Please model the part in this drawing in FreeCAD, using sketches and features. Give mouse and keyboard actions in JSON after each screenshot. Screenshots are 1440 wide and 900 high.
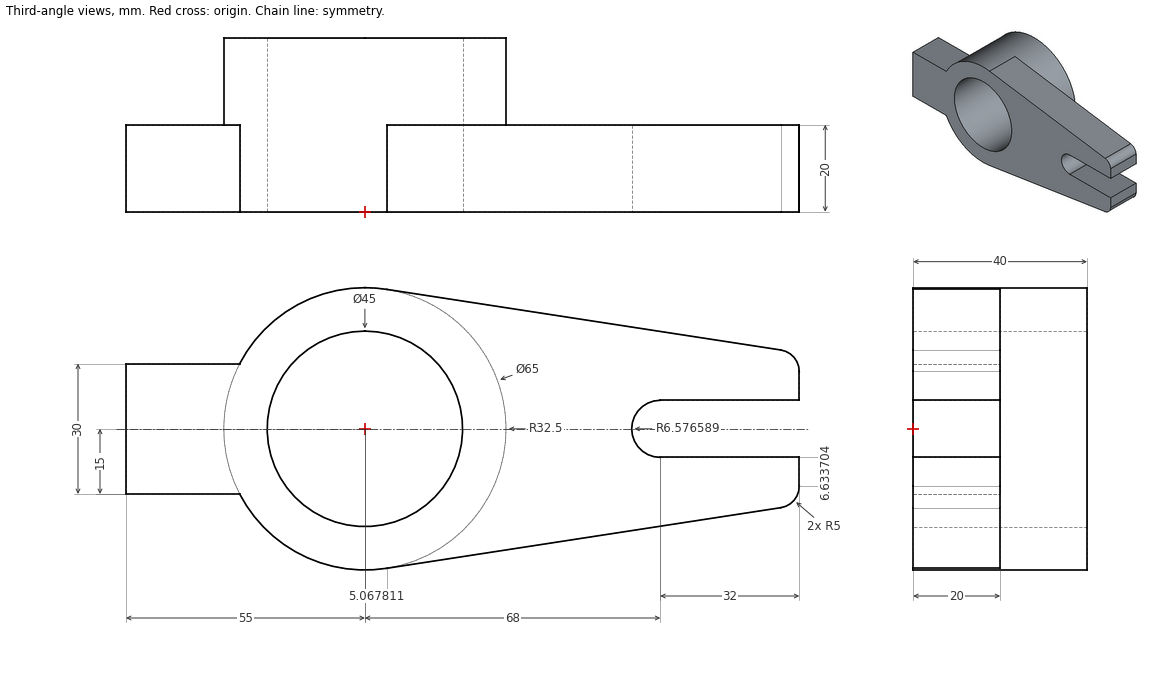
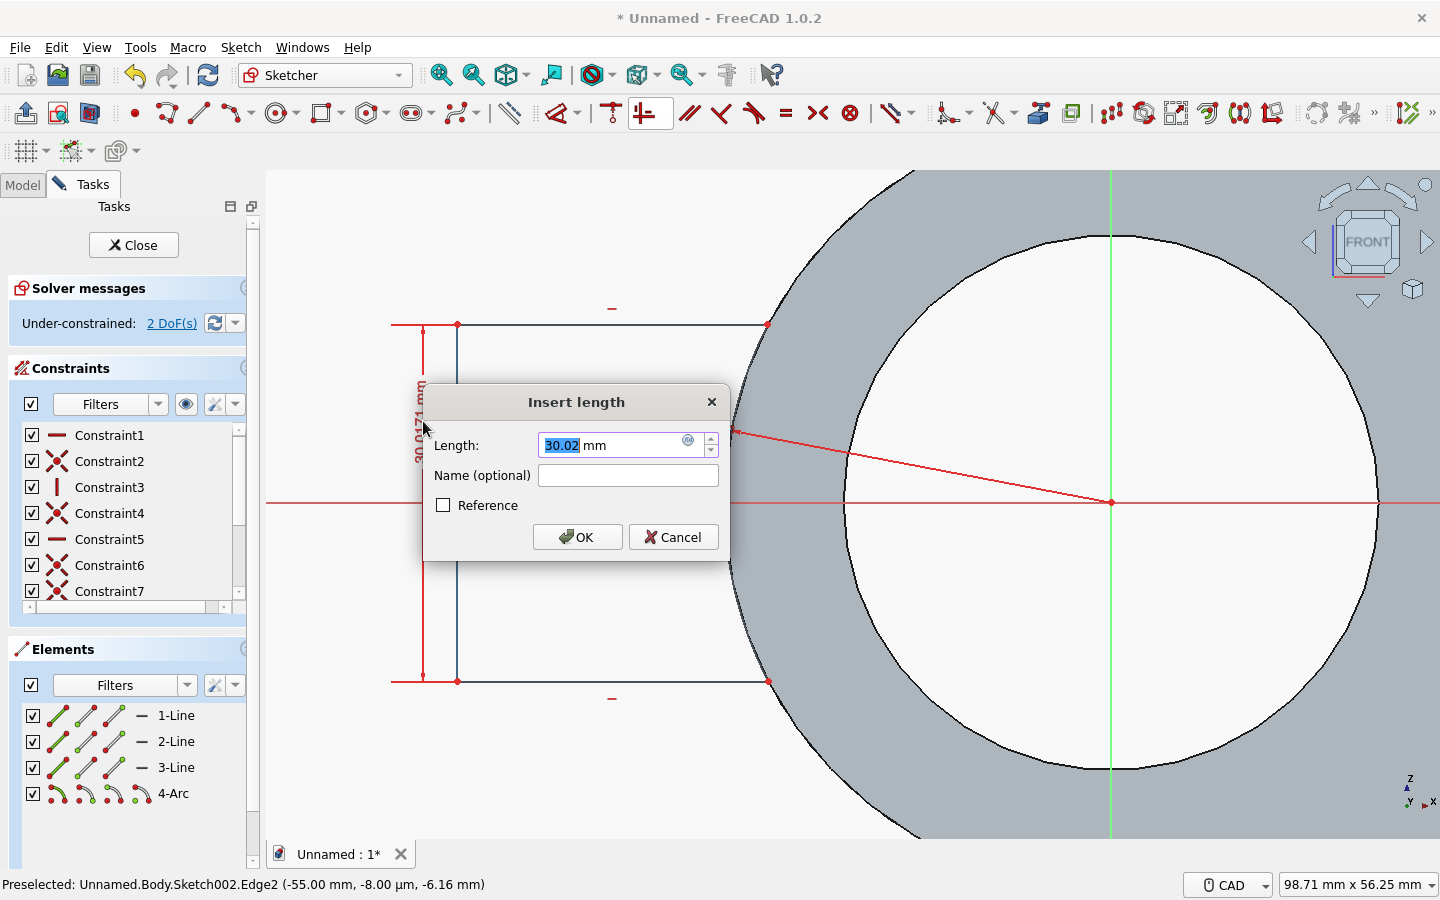
{"action": "type", "text": "30"}
{"action": "key", "text": "Return"}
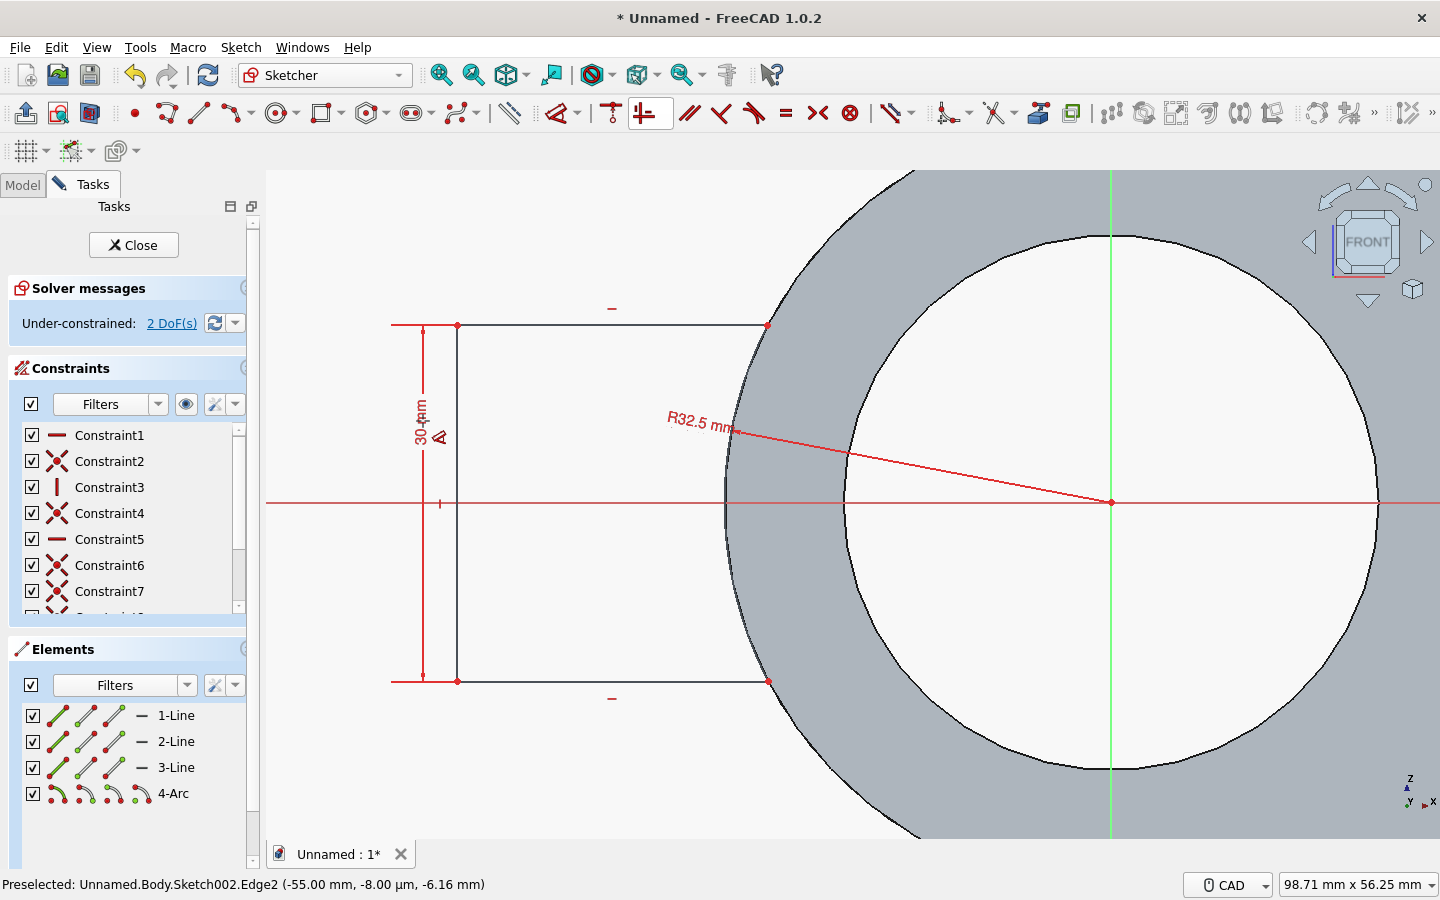
{"action": "left_click", "coordinate": [769, 682]}
{"action": "left_click", "coordinate": [1145, 592]}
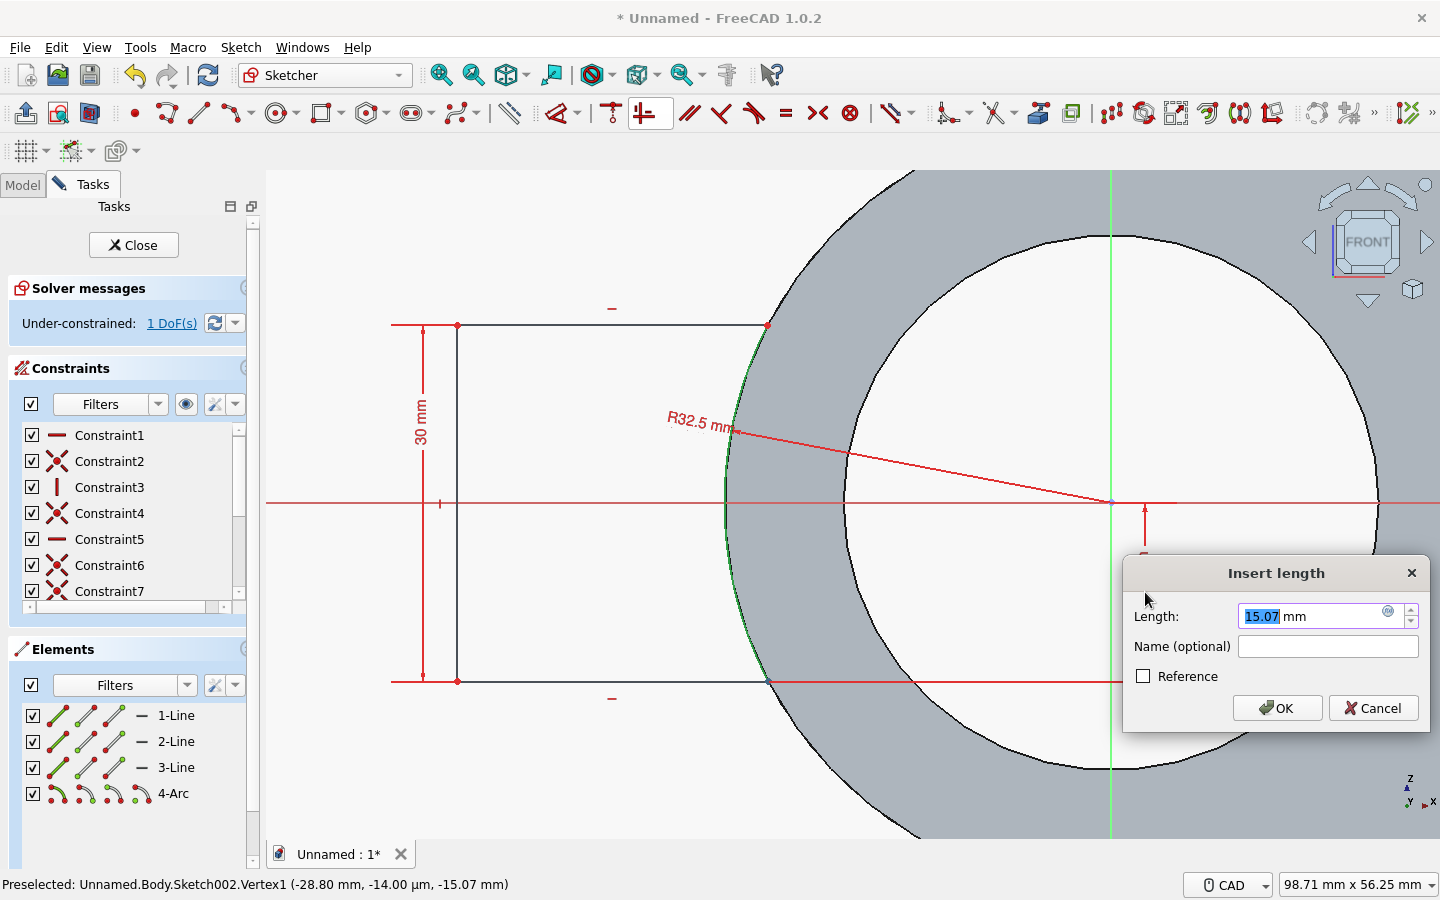
{"action": "type", "text": "15"}
{"action": "key", "text": "Return"}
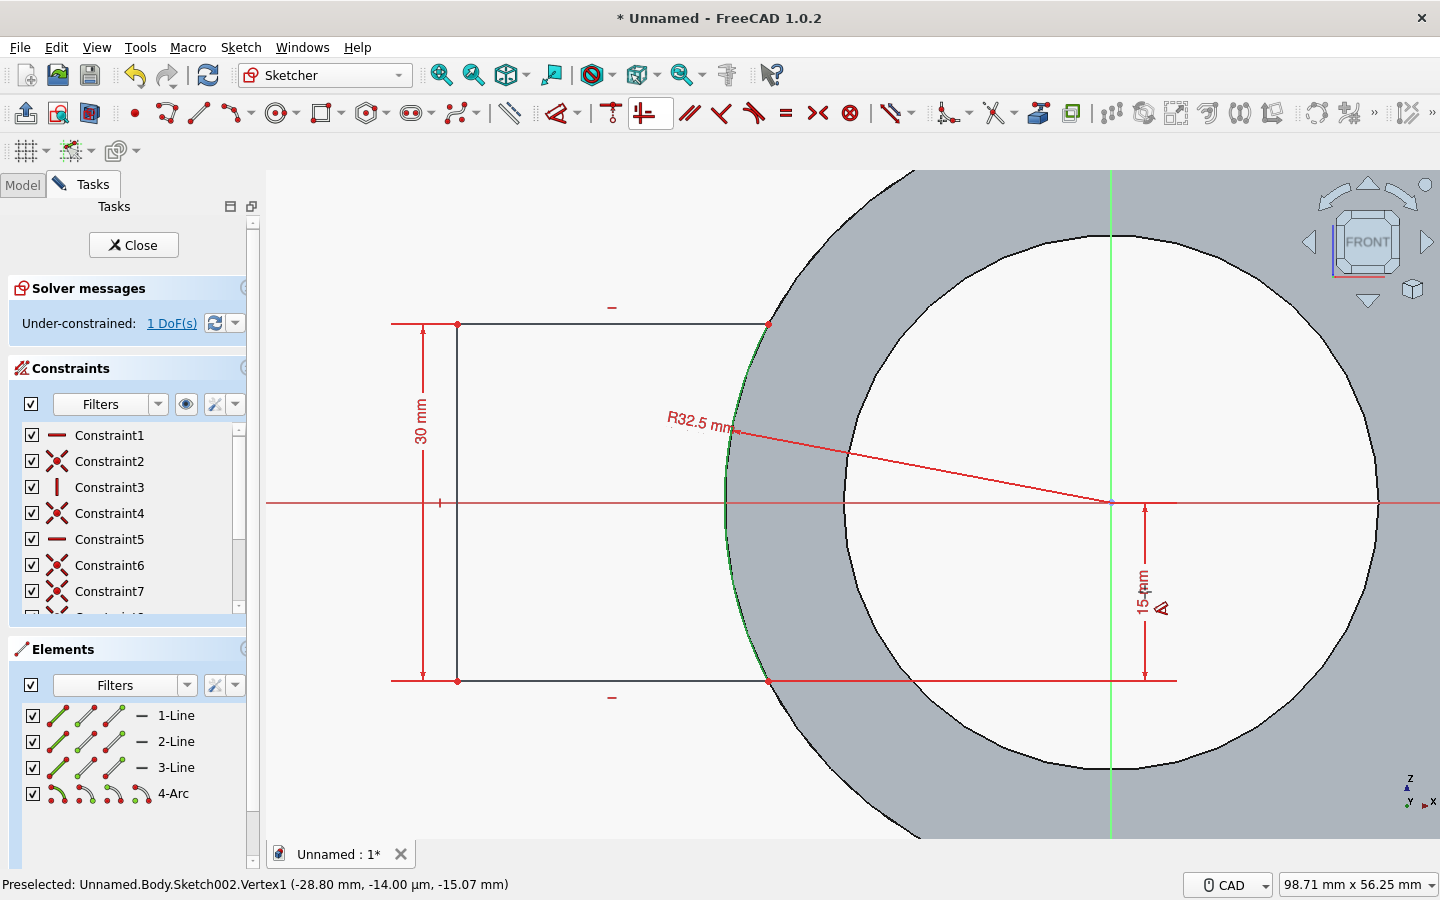
{"action": "left_click", "coordinate": [457, 681]}
{"action": "left_click", "coordinate": [784, 715]}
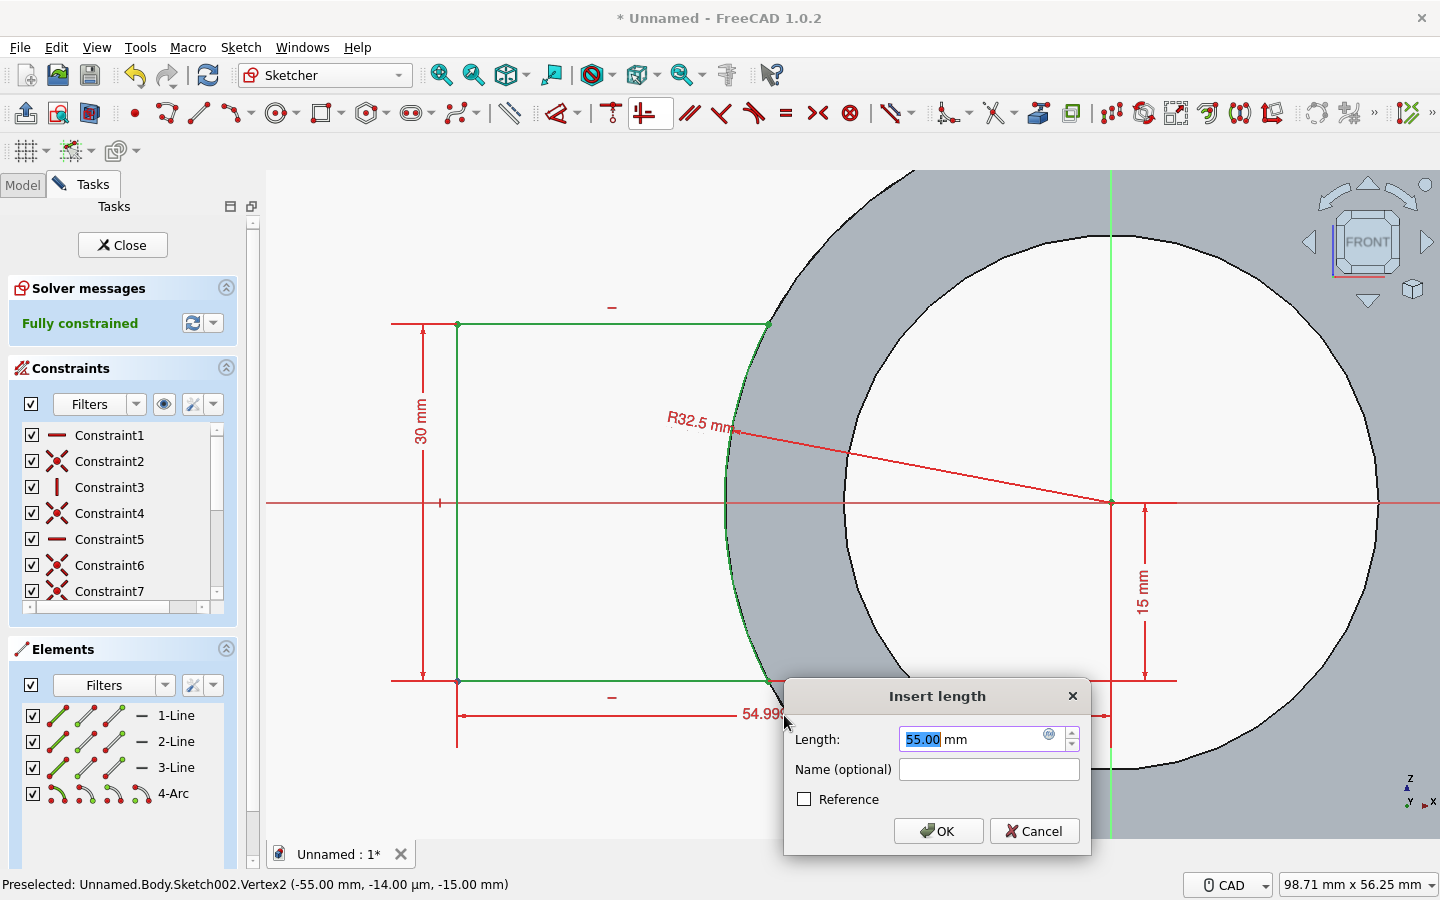
{"action": "type", "text": "55"}
{"action": "key", "text": "Return"}
{"action": "key", "text": "Escape"}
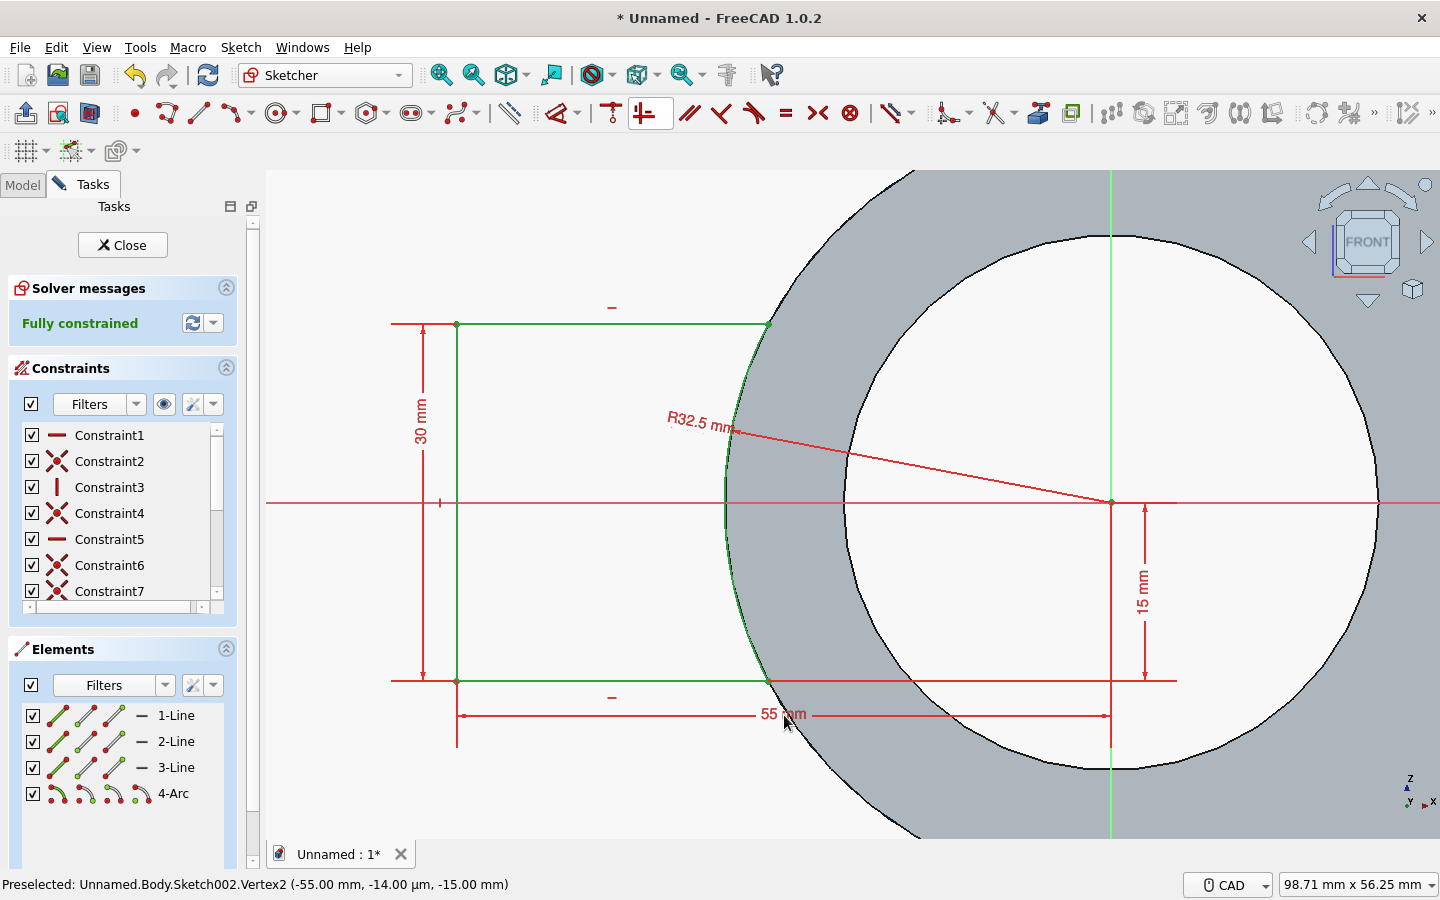
{"action": "left_click", "coordinate": [123, 245]}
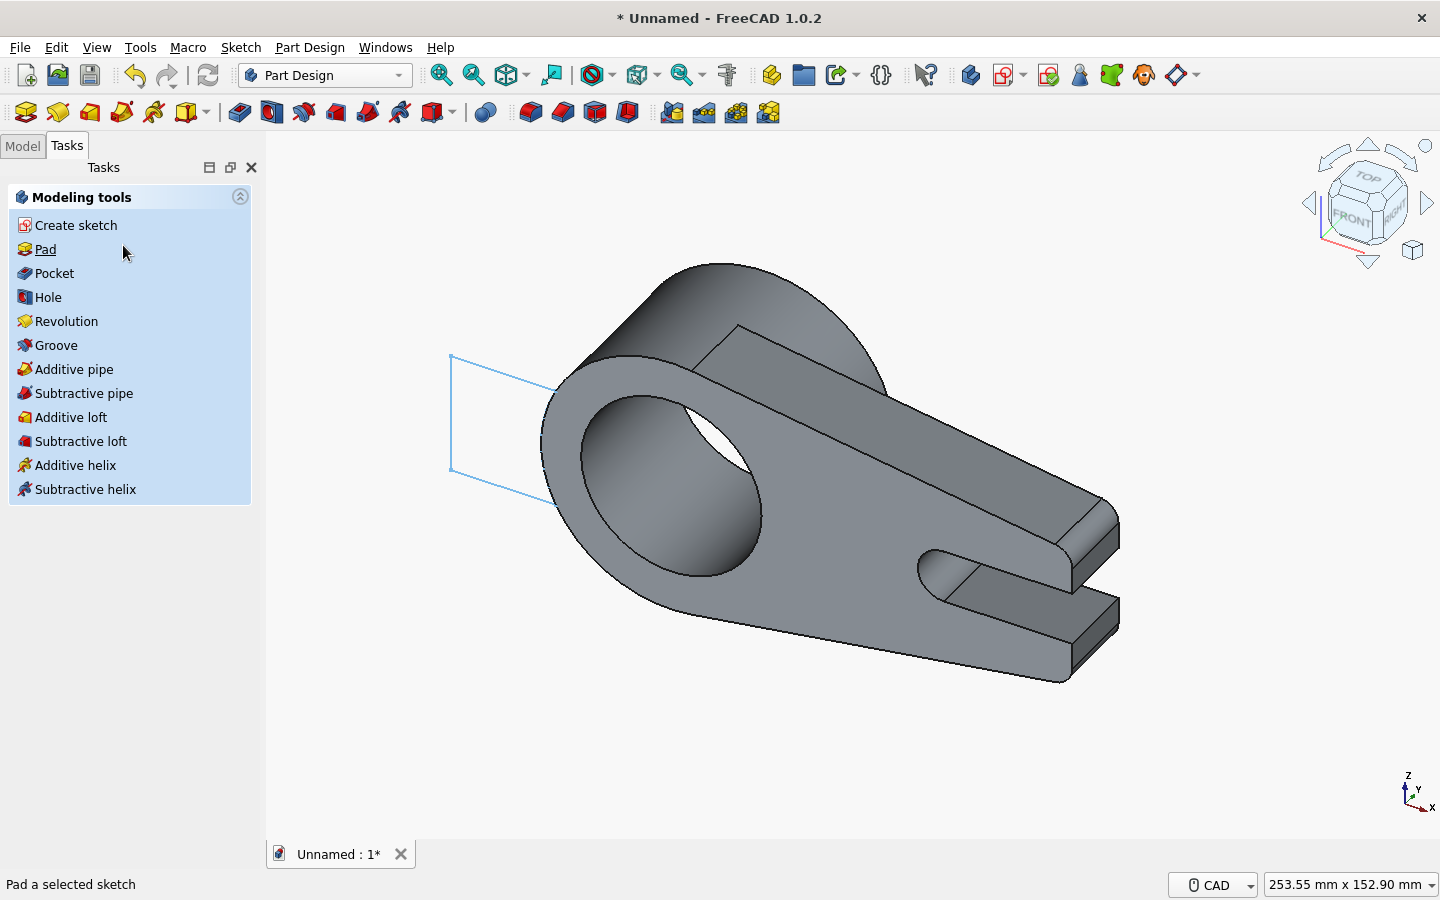
{"action": "left_click", "coordinate": [26, 112]}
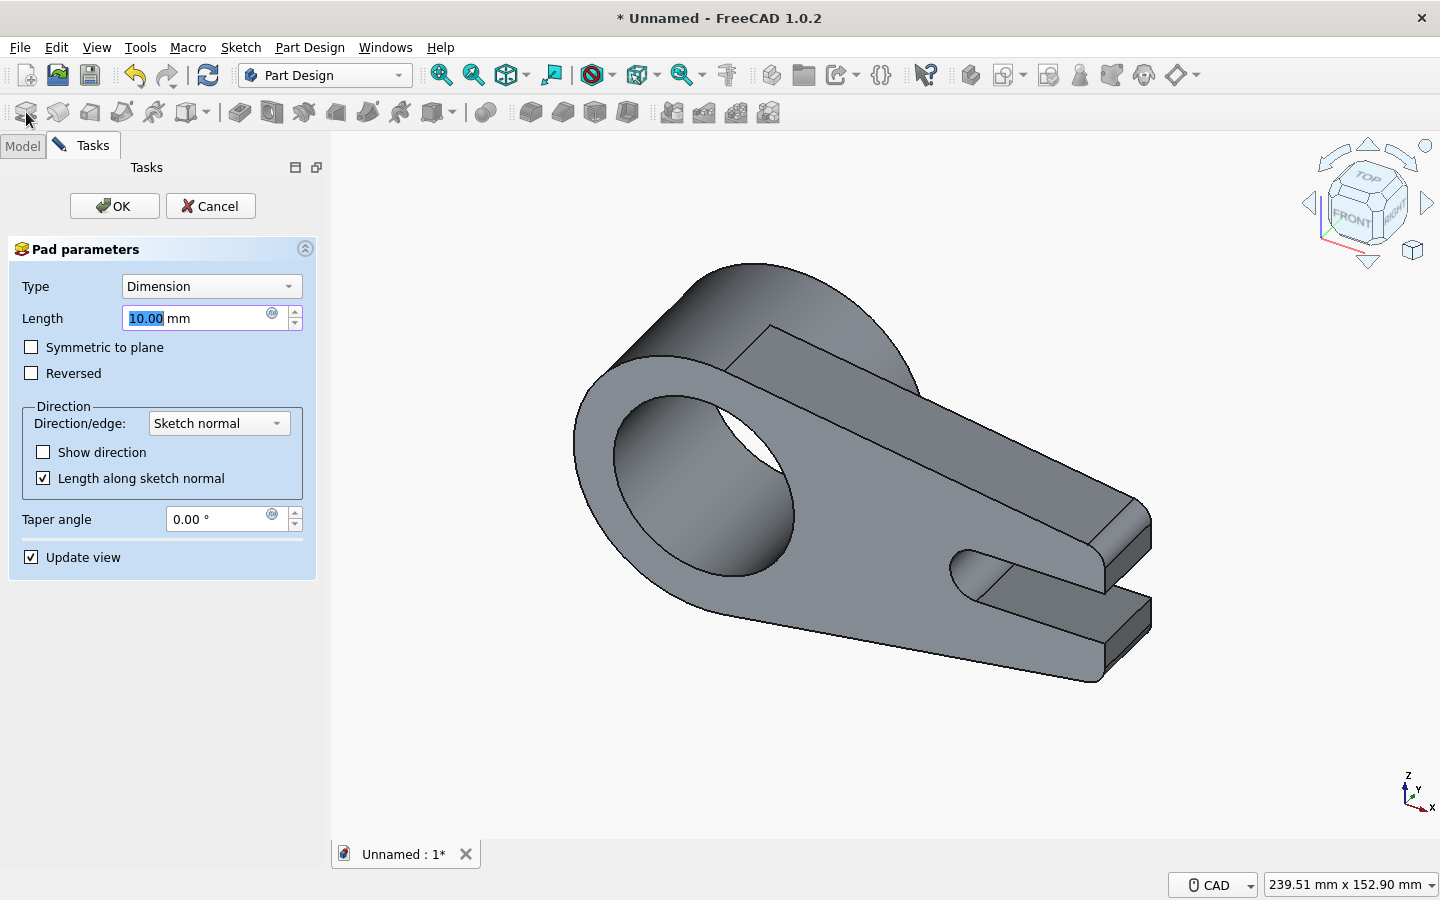
{"action": "type", "text": "20"}
{"action": "key", "text": "Tab"}